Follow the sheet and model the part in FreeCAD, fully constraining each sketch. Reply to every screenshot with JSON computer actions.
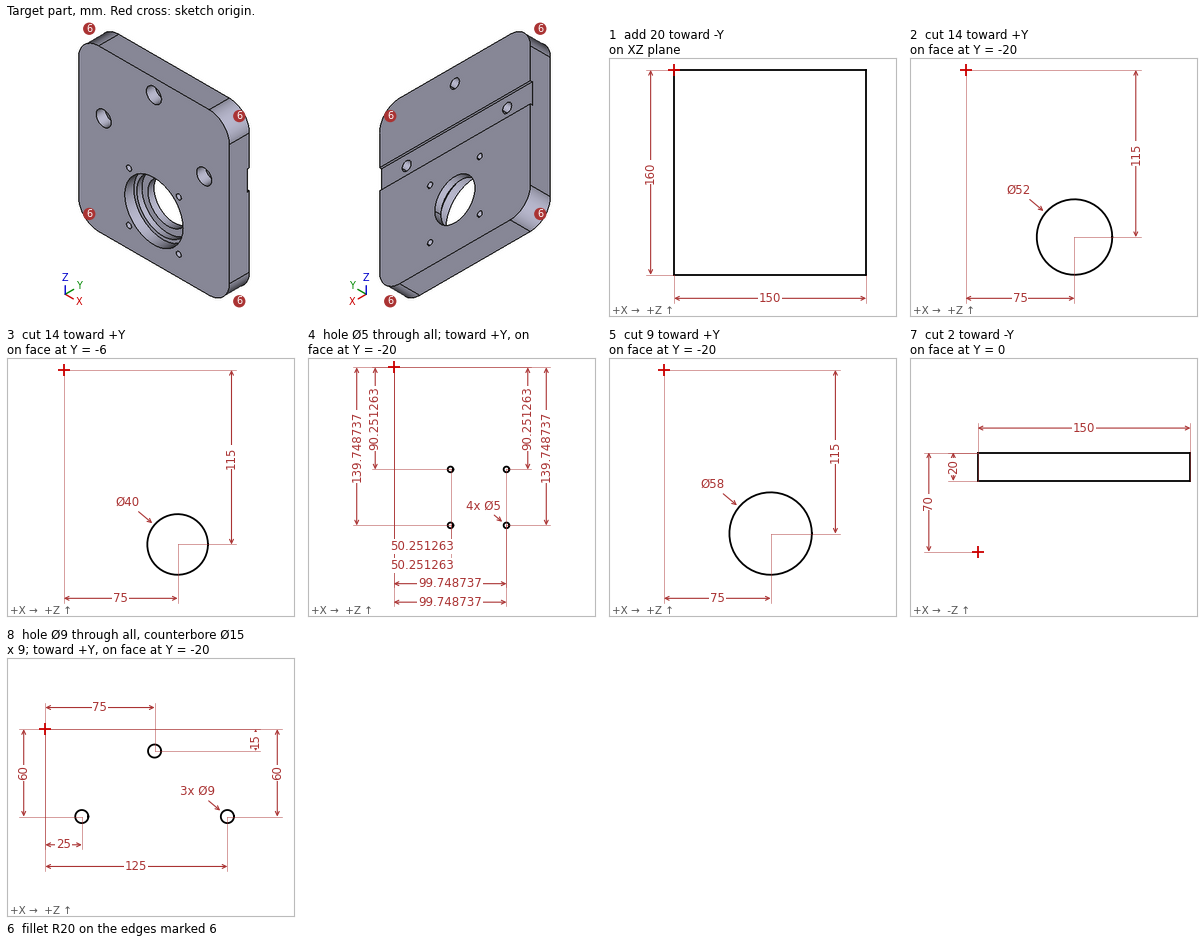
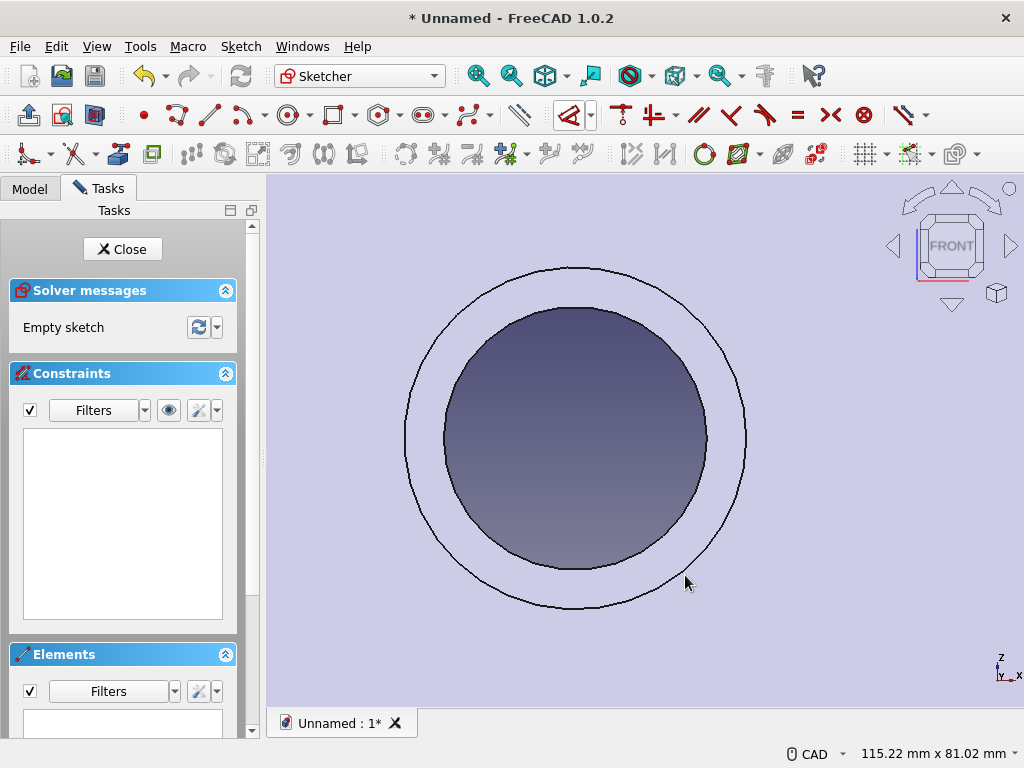
{"action": "left_click", "coordinate": [288, 116]}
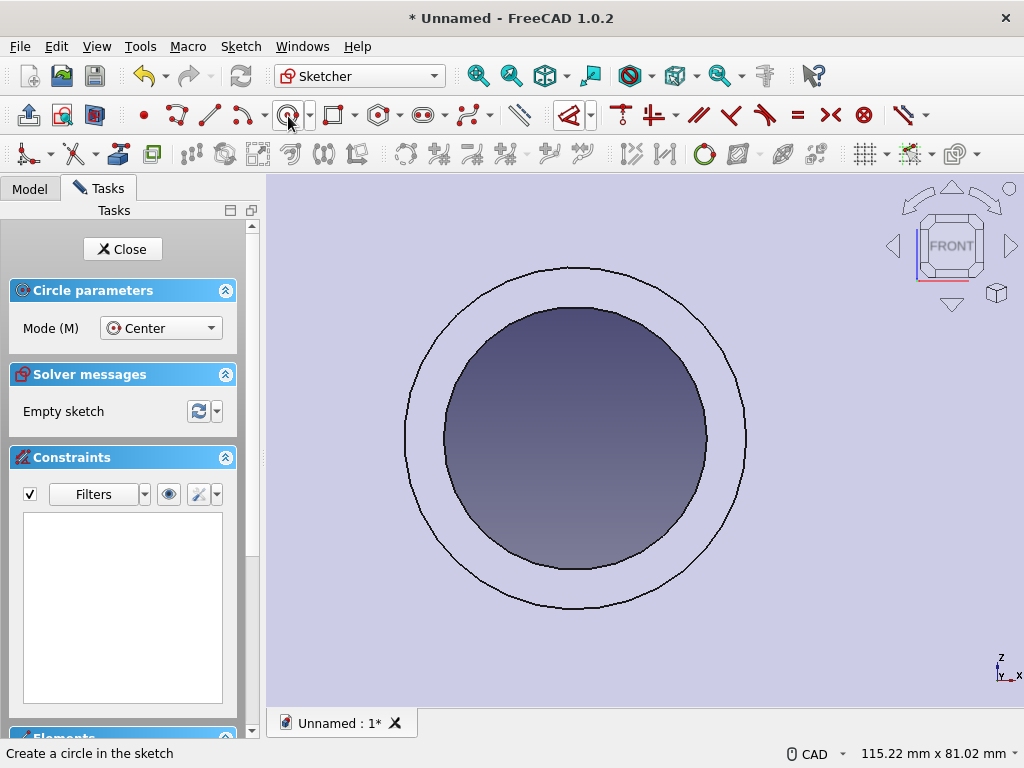
{"action": "scroll", "coordinate": [738, 601], "scroll_direction": "up", "scroll_amount": 2}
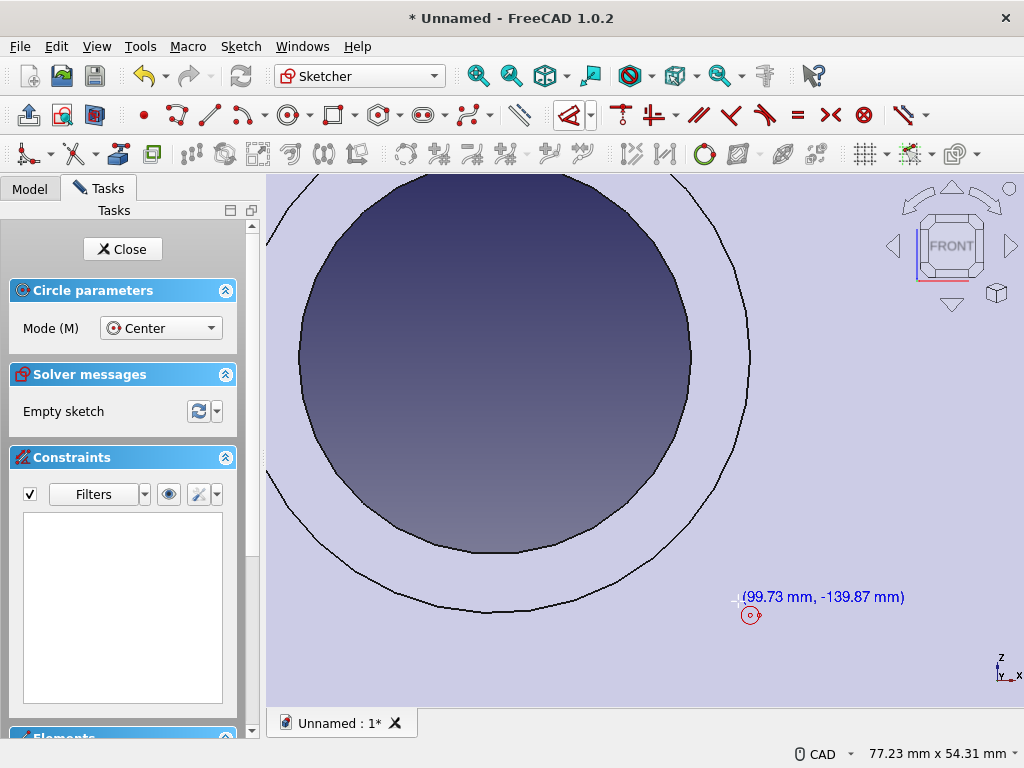
{"action": "left_click", "coordinate": [738, 601]}
{"action": "left_click", "coordinate": [755, 584]}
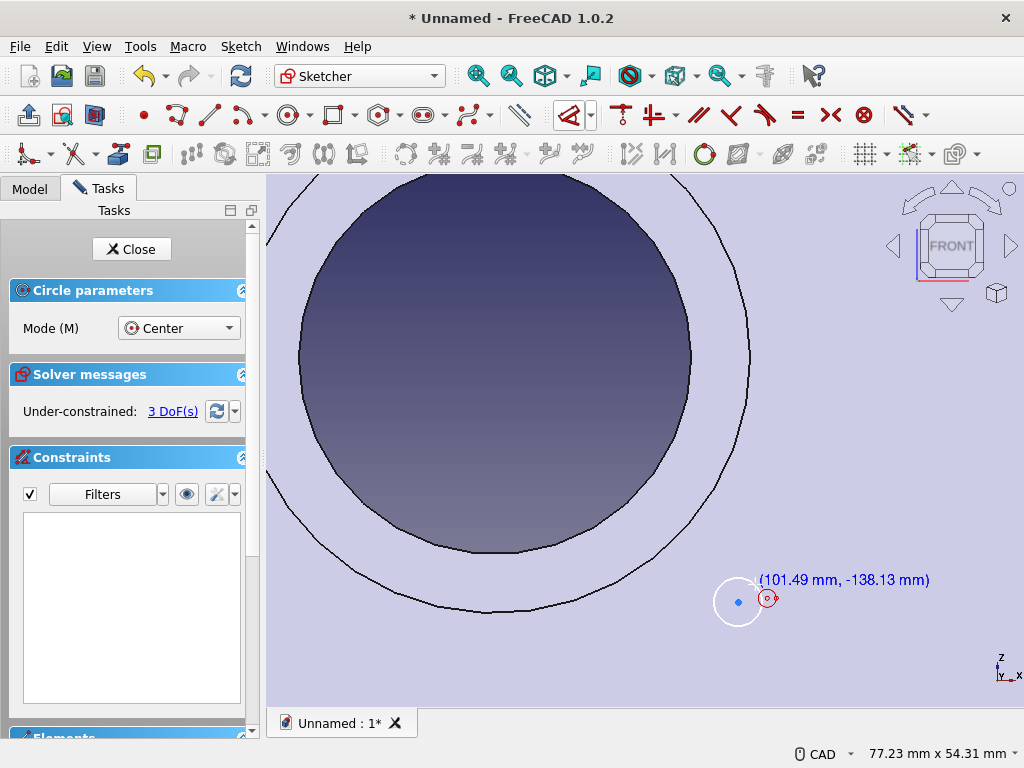
{"action": "scroll", "coordinate": [742, 608], "scroll_direction": "down", "scroll_amount": 2}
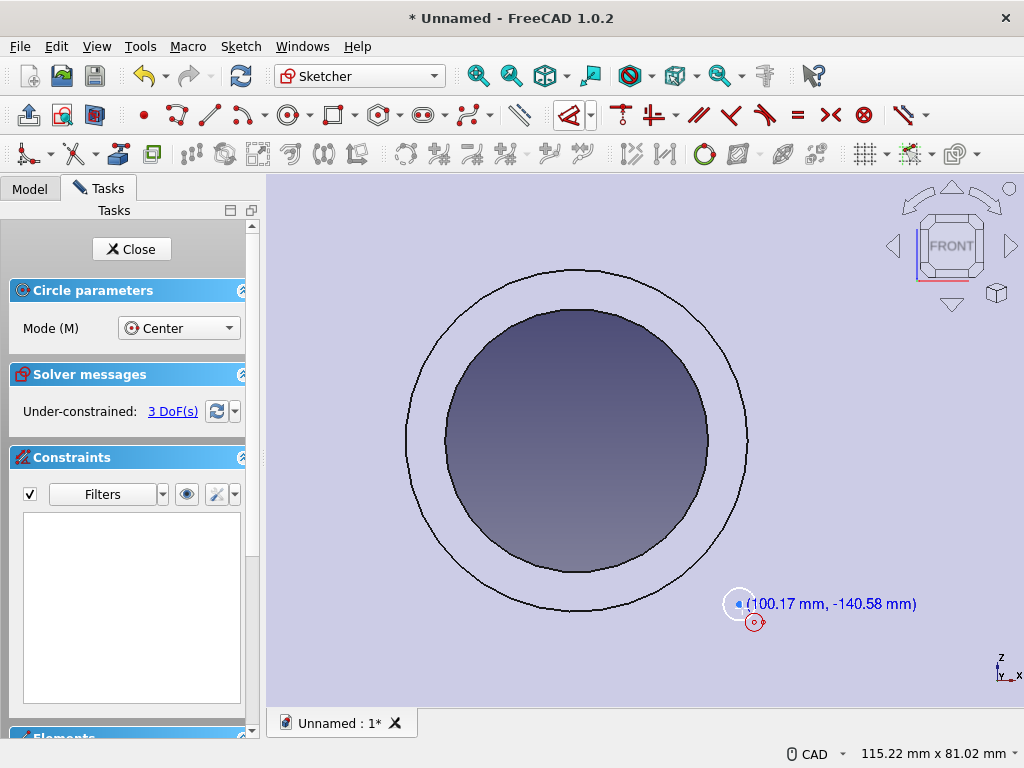
{"action": "scroll", "coordinate": [414, 603], "scroll_direction": "up", "scroll_amount": 2}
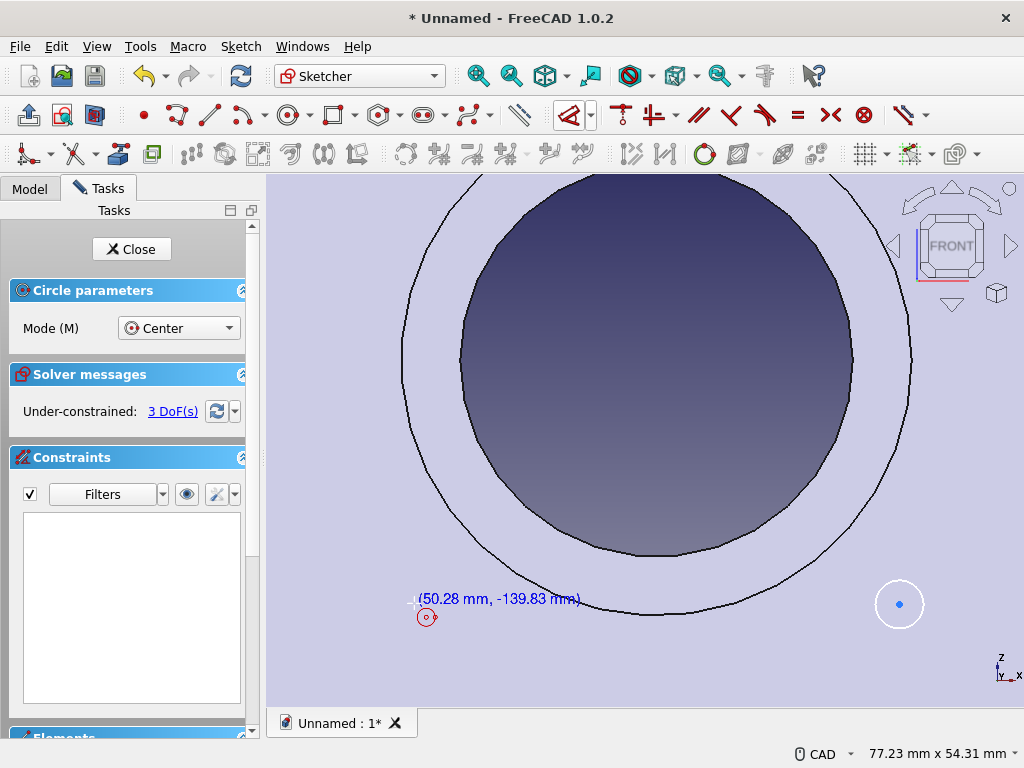
{"action": "left_click", "coordinate": [414, 603]}
{"action": "left_click", "coordinate": [431, 586]}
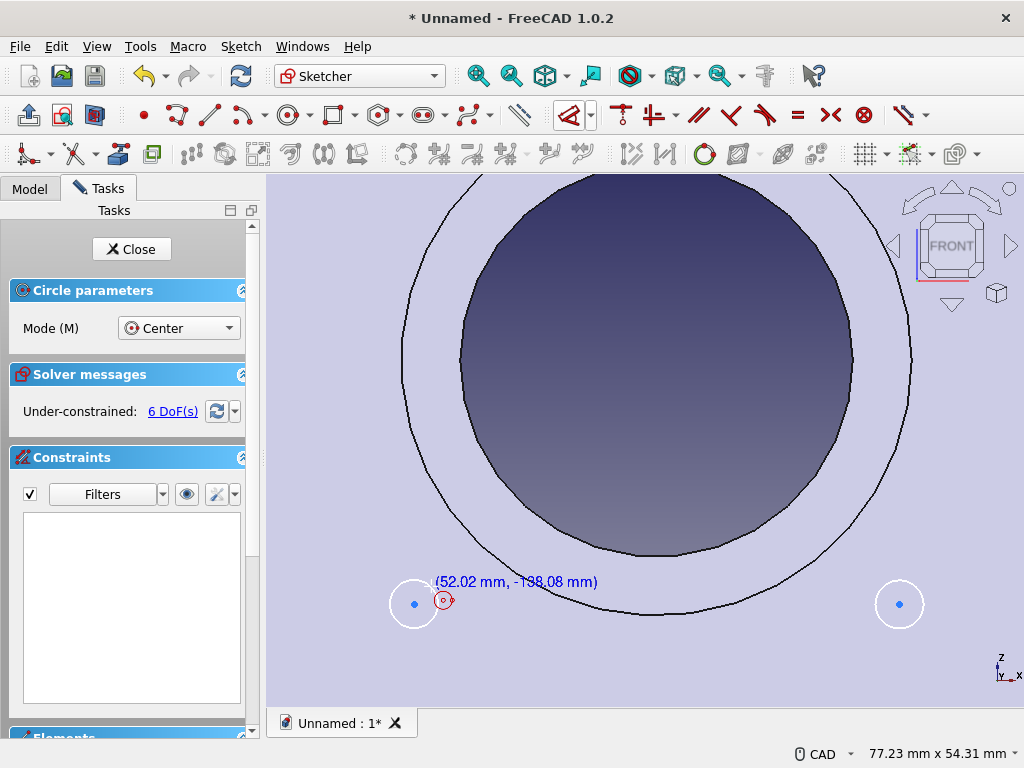
{"action": "scroll", "coordinate": [414, 603], "scroll_direction": "down", "scroll_amount": 2}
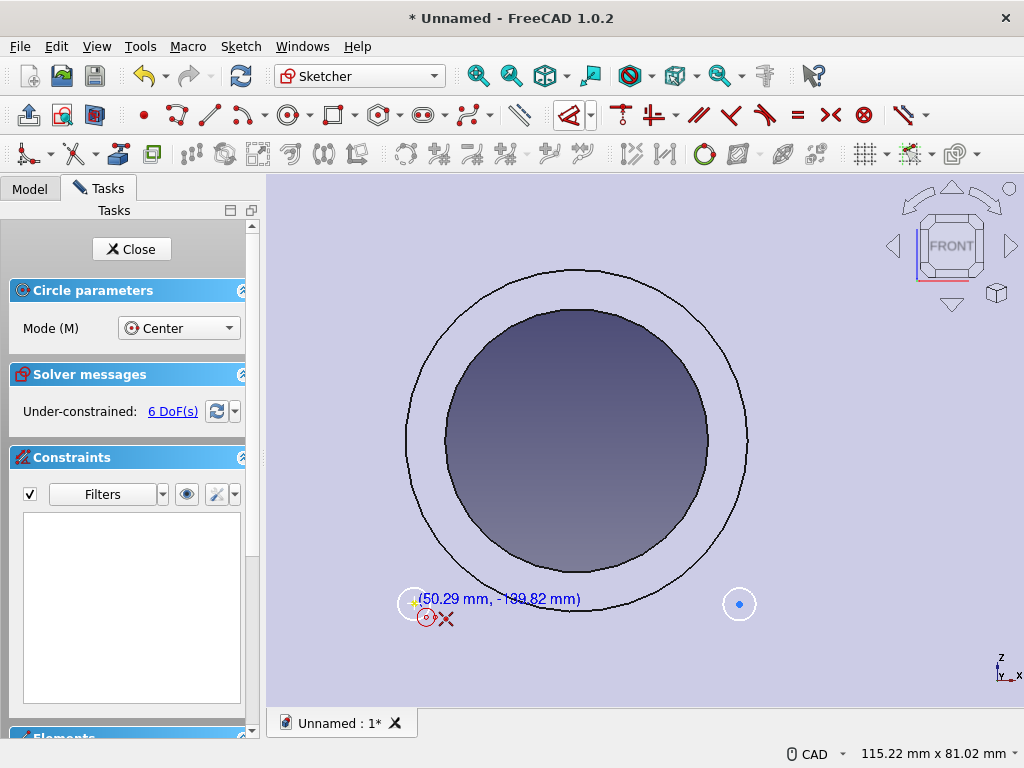
{"action": "scroll", "coordinate": [414, 278], "scroll_direction": "up", "scroll_amount": 2}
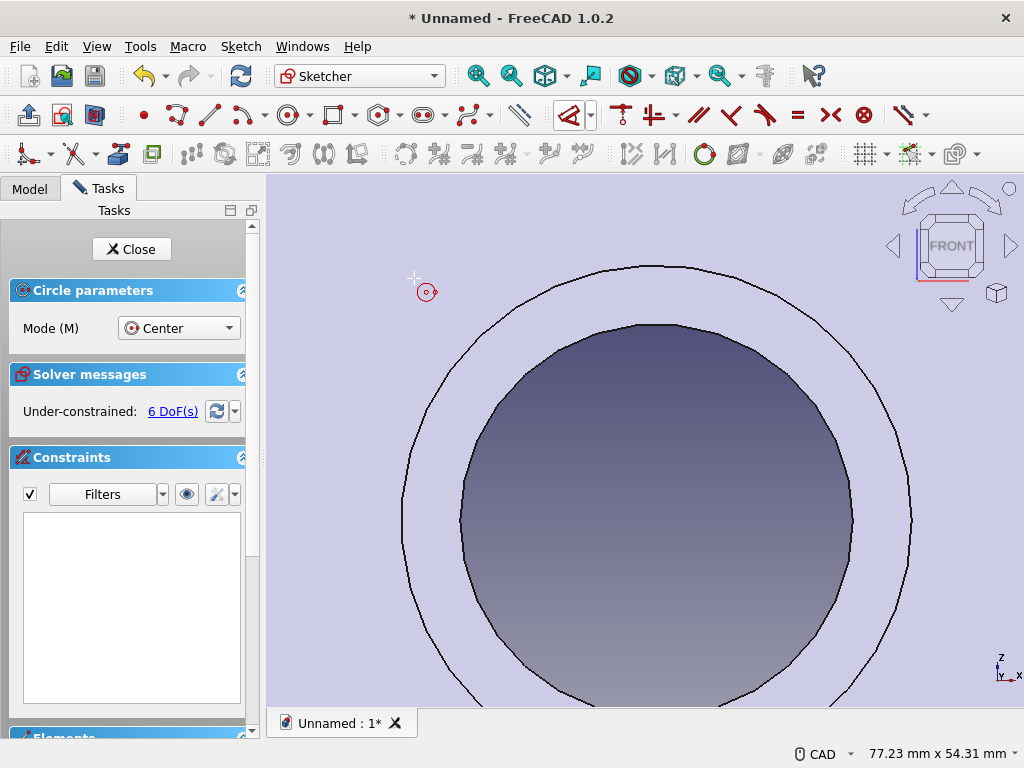
{"action": "left_click", "coordinate": [414, 278]}
{"action": "left_click", "coordinate": [431, 260]}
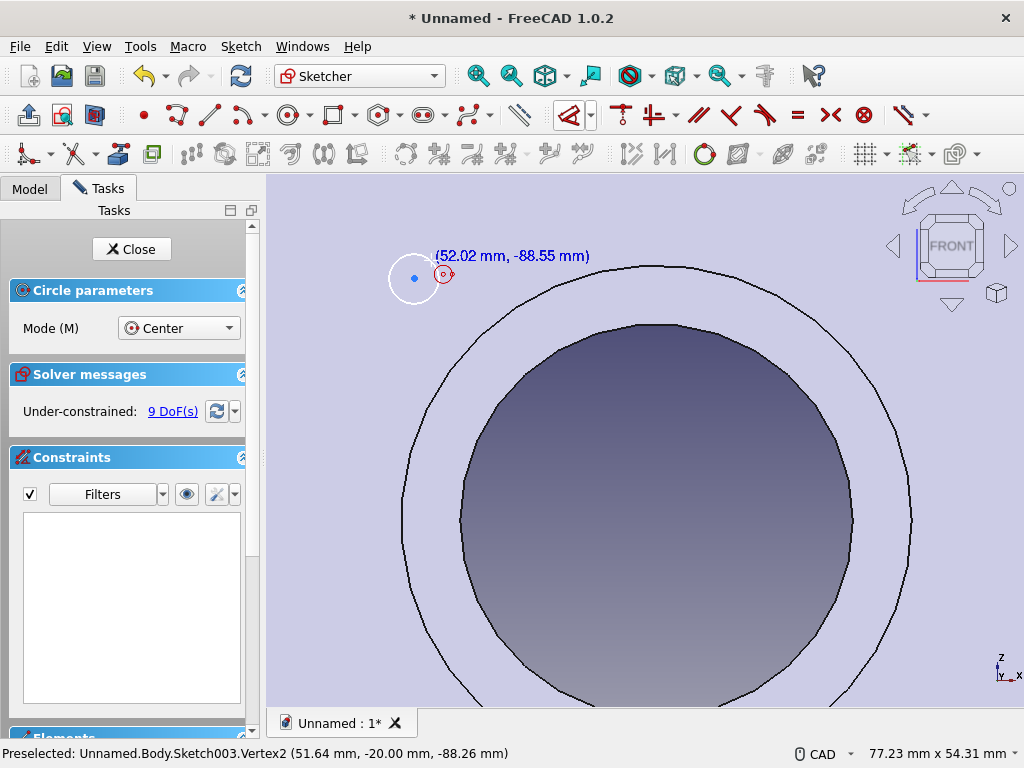
{"action": "scroll", "coordinate": [414, 278], "scroll_direction": "down", "scroll_amount": 2}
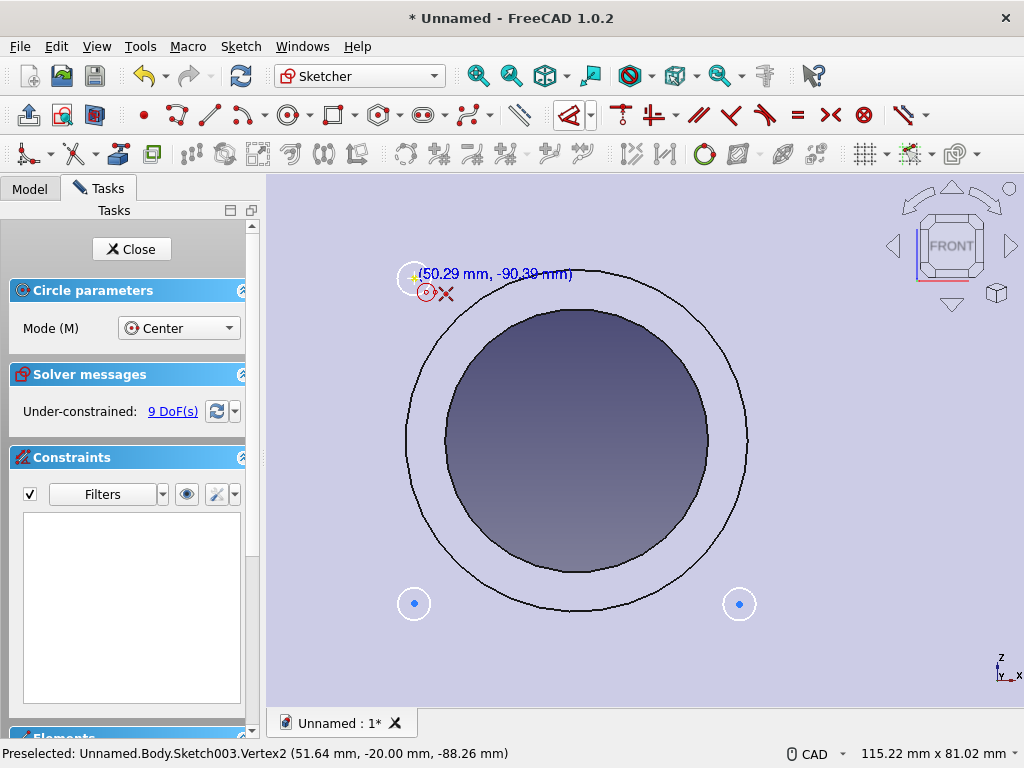
{"action": "scroll", "coordinate": [739, 278], "scroll_direction": "up", "scroll_amount": 2}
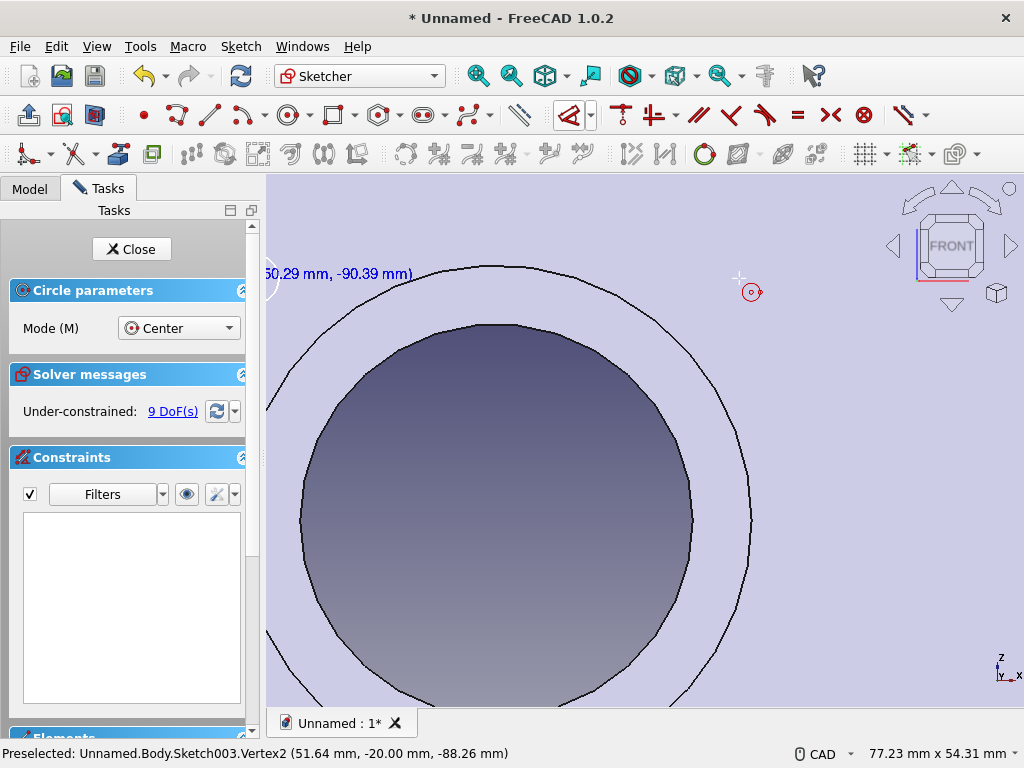
{"action": "left_click", "coordinate": [739, 278]}
{"action": "left_click", "coordinate": [757, 260]}
{"action": "key", "text": "Escape"}